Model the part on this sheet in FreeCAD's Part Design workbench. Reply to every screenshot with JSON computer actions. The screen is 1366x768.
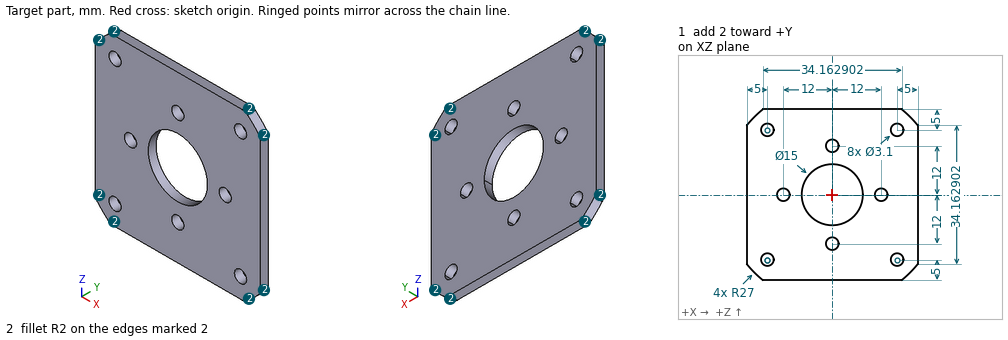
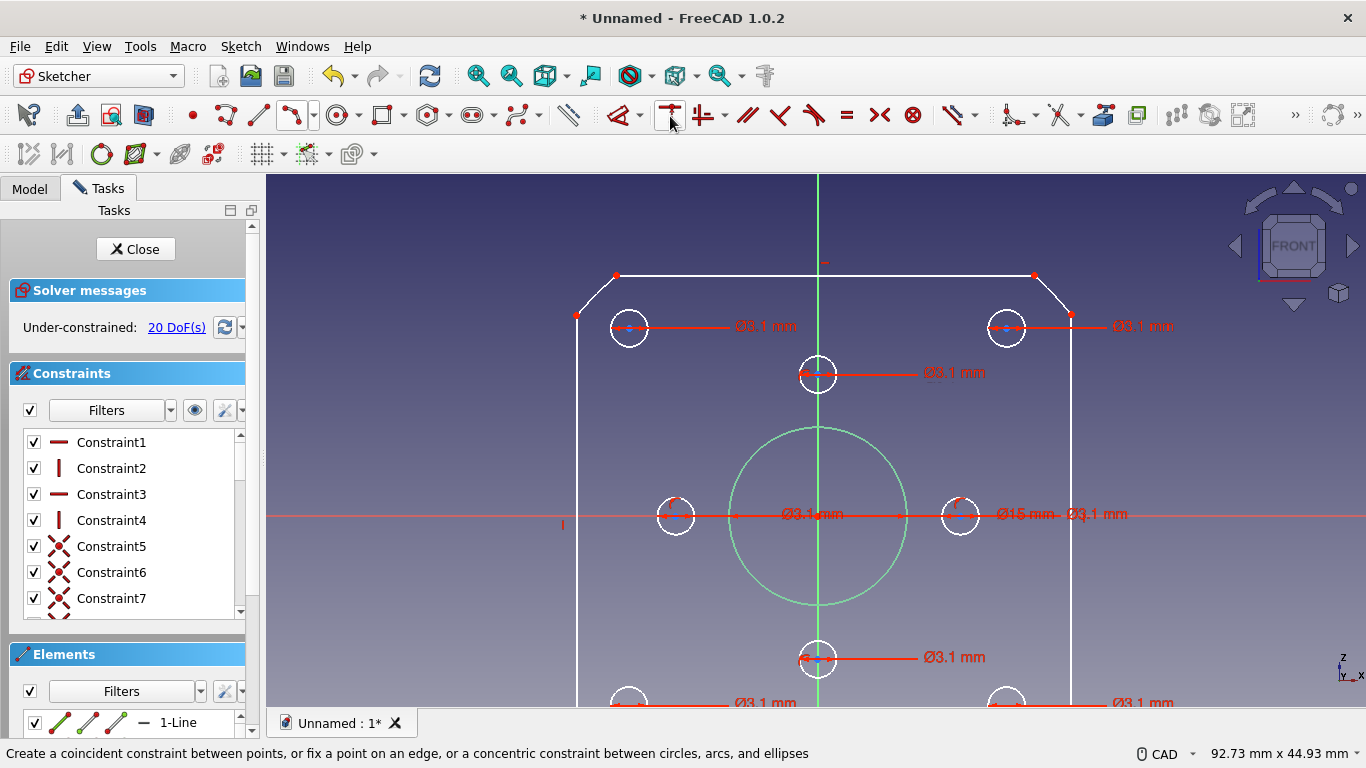
{"action": "left_click", "coordinate": [1061, 302]}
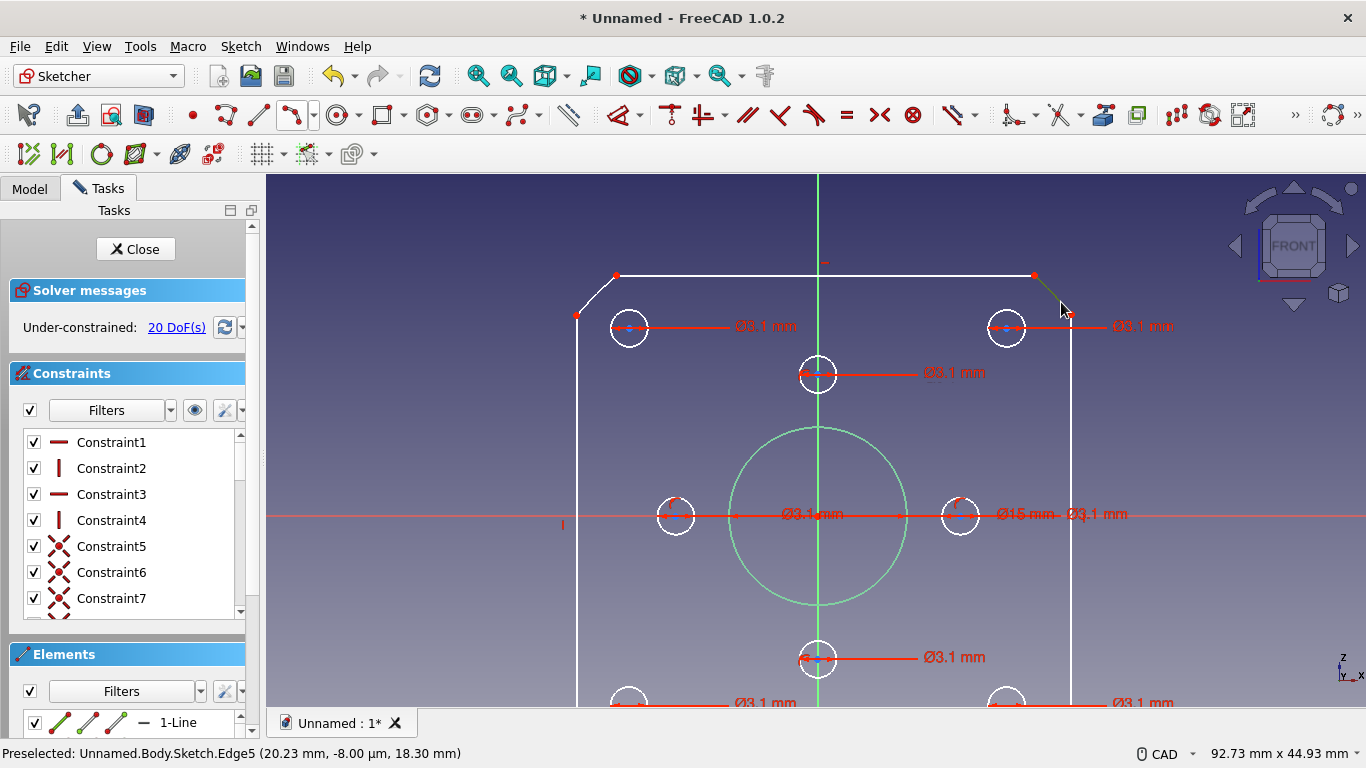
{"action": "scroll", "coordinate": [604, 287], "scroll_direction": "down", "scroll_amount": 2}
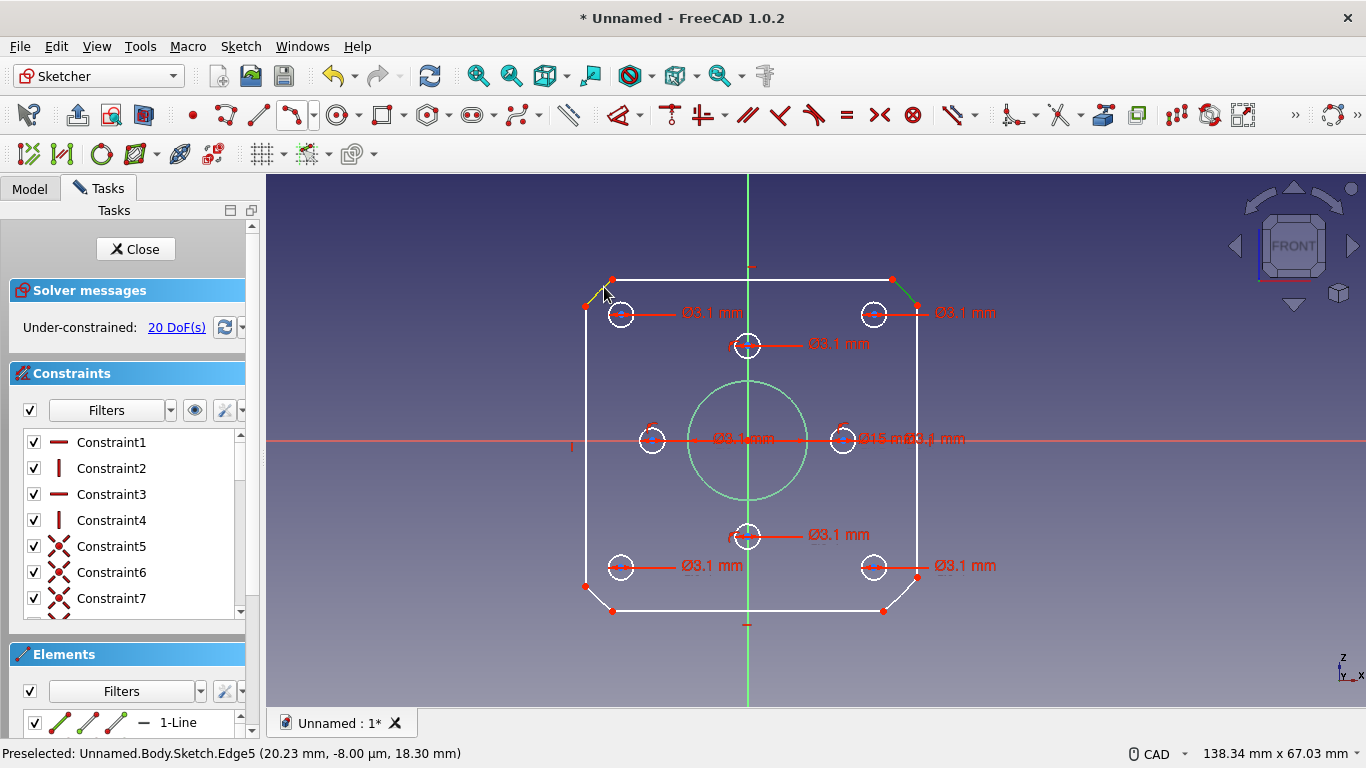
{"action": "left_click", "coordinate": [894, 602]}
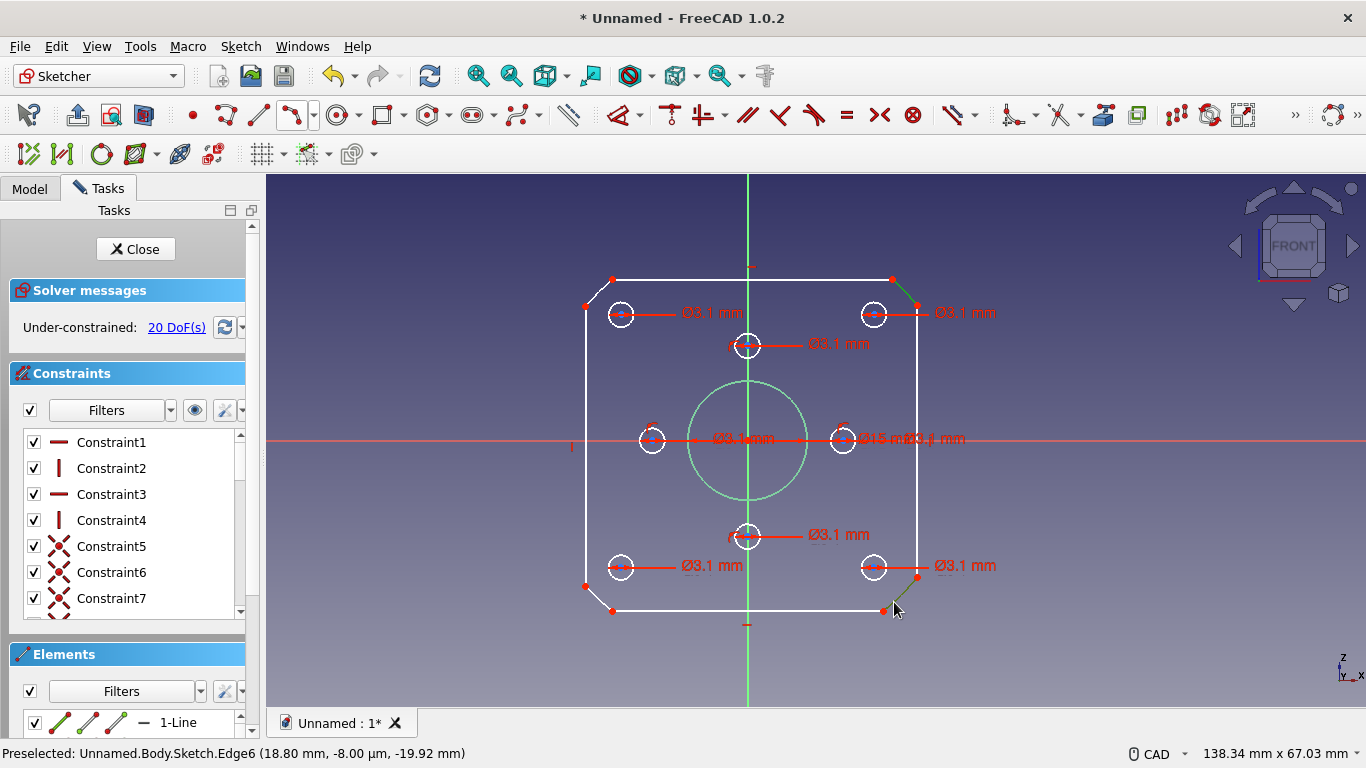
{"action": "scroll", "coordinate": [593, 594], "scroll_direction": "up", "scroll_amount": 2}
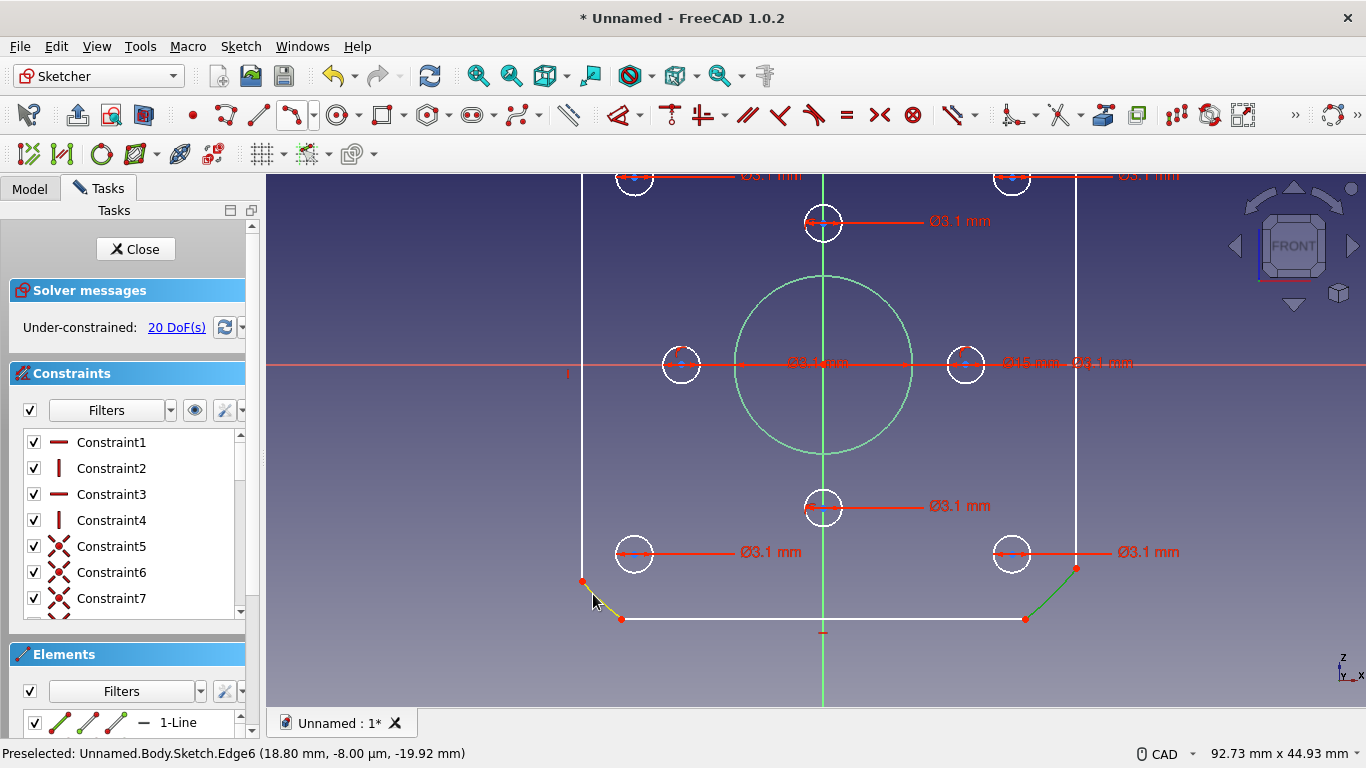
{"action": "left_click", "coordinate": [593, 594]}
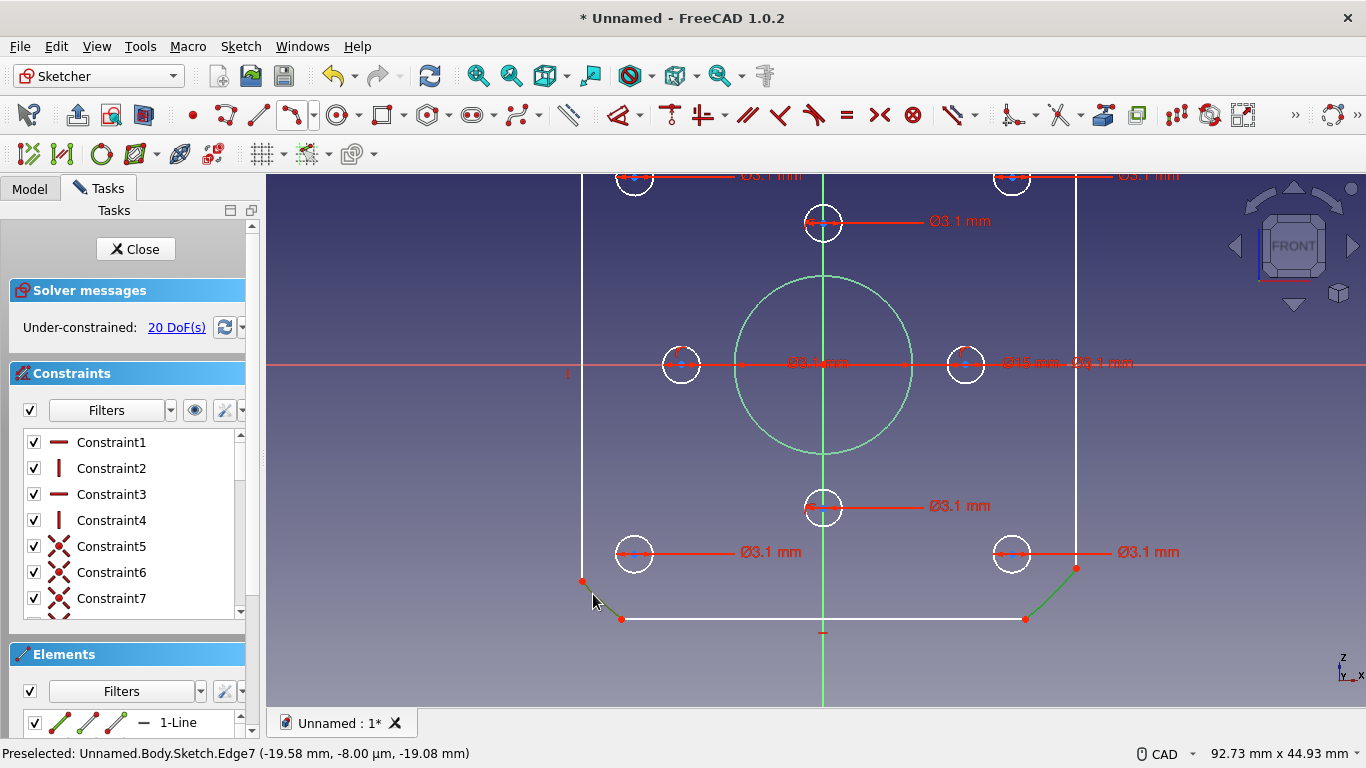
{"action": "scroll", "coordinate": [593, 594], "scroll_direction": "down", "scroll_amount": 2}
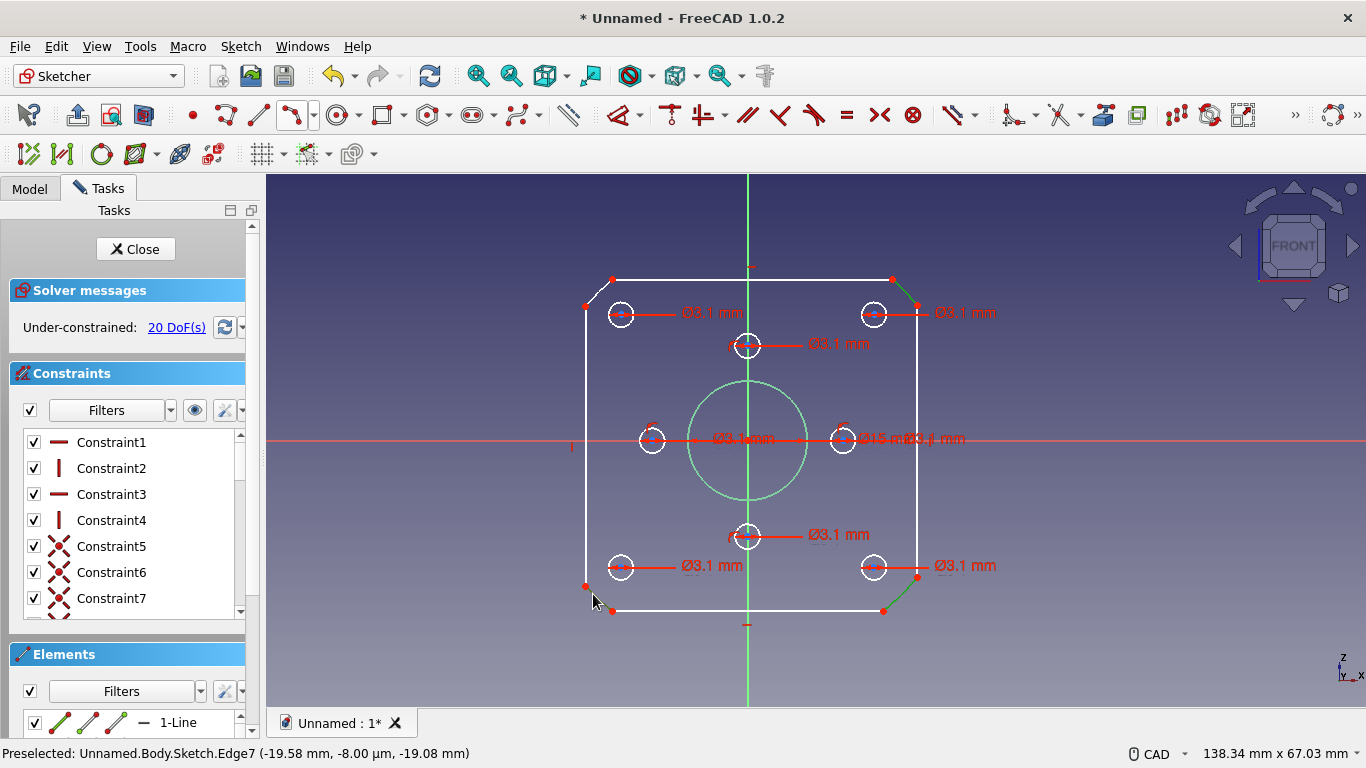
{"action": "left_click", "coordinate": [604, 287]}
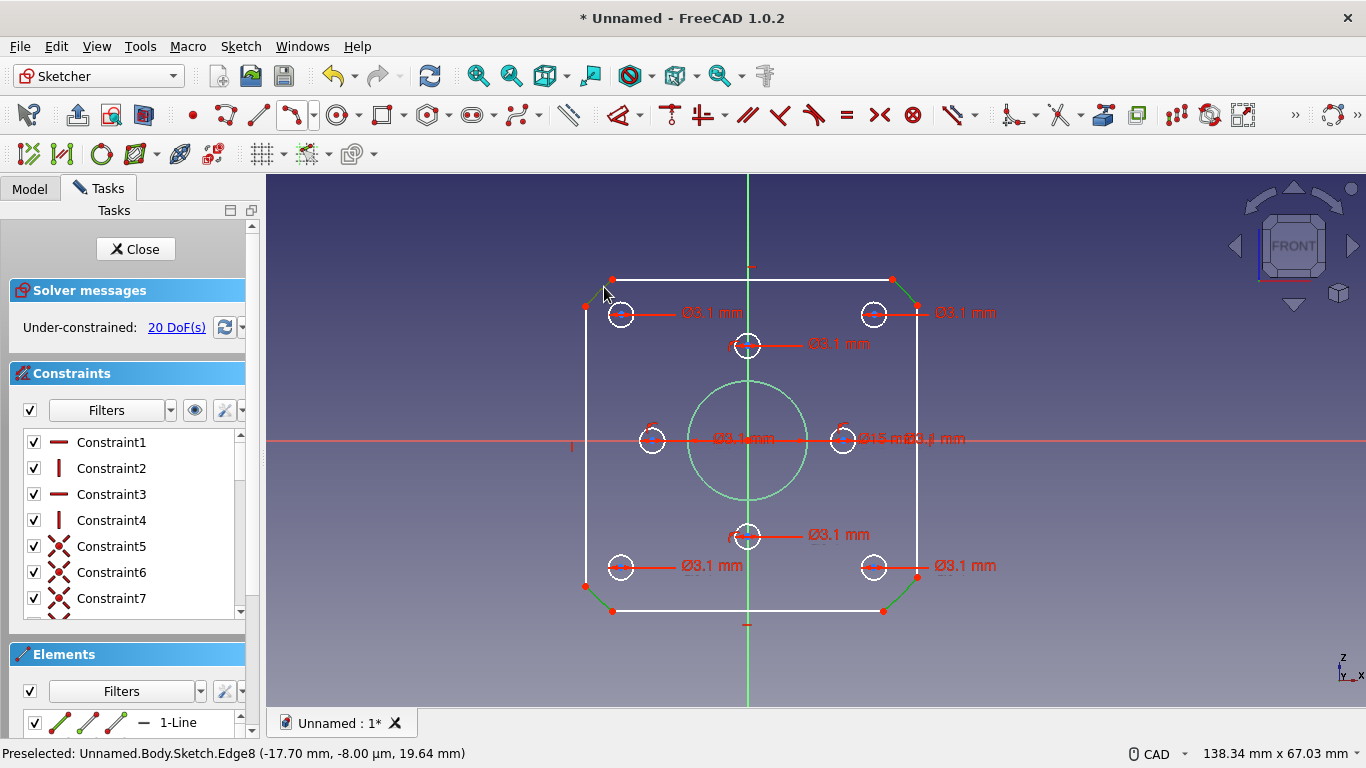
{"action": "left_click", "coordinate": [847, 116]}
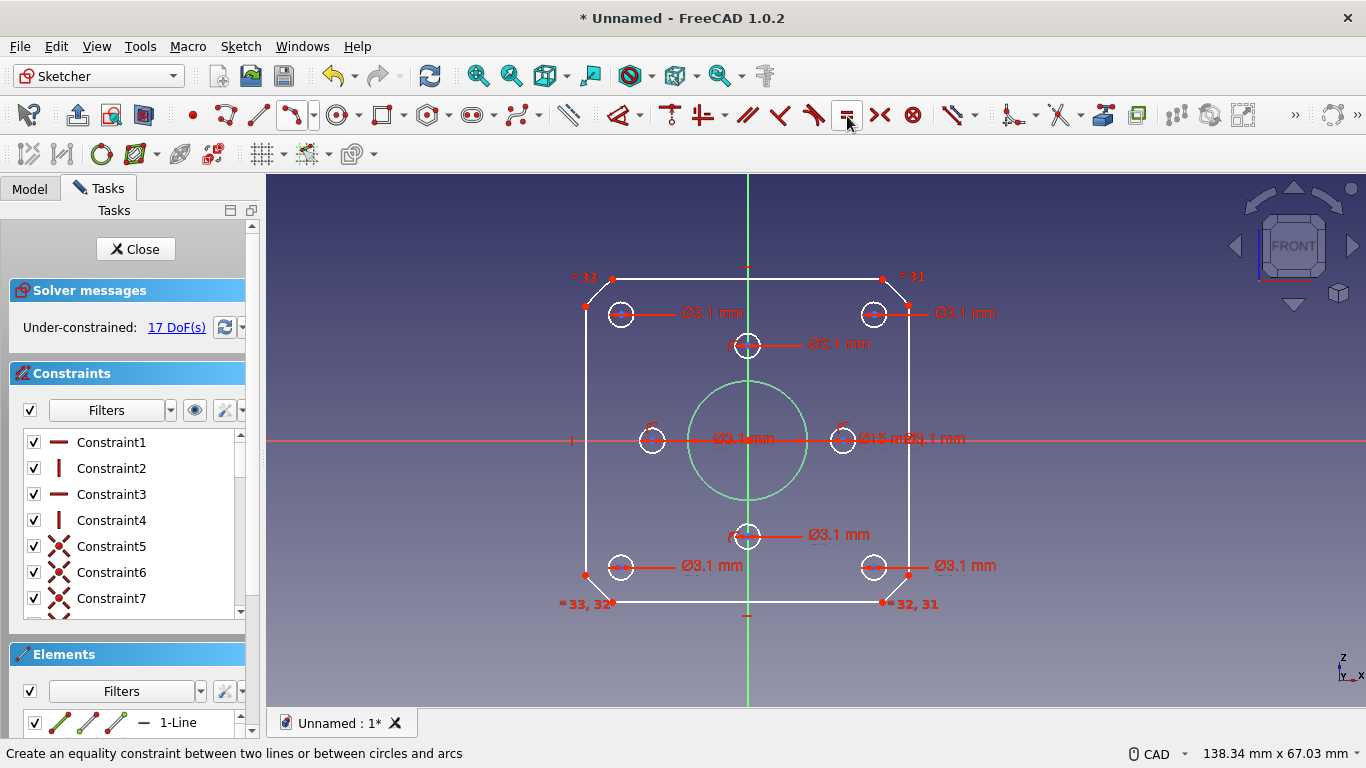
{"action": "left_click", "coordinate": [874, 315]}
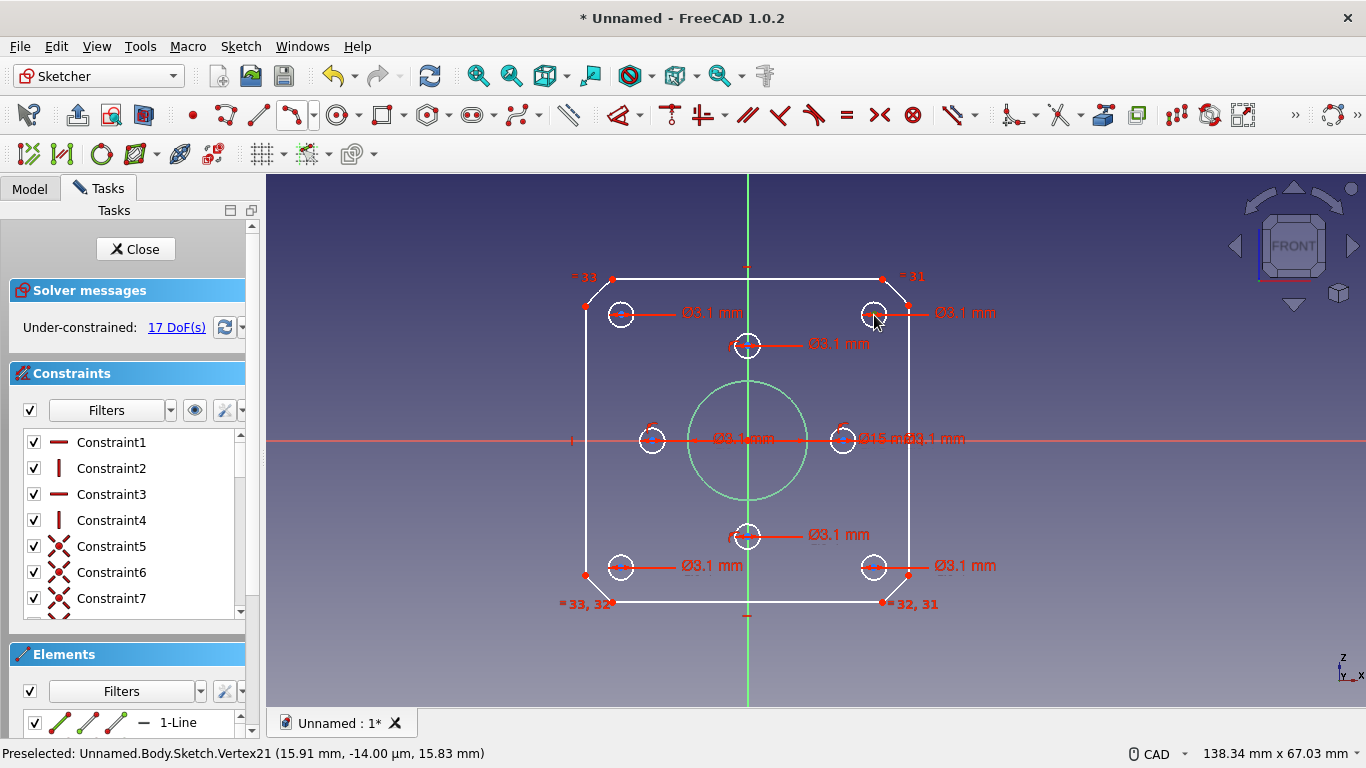
{"action": "left_click", "coordinate": [621, 315]}